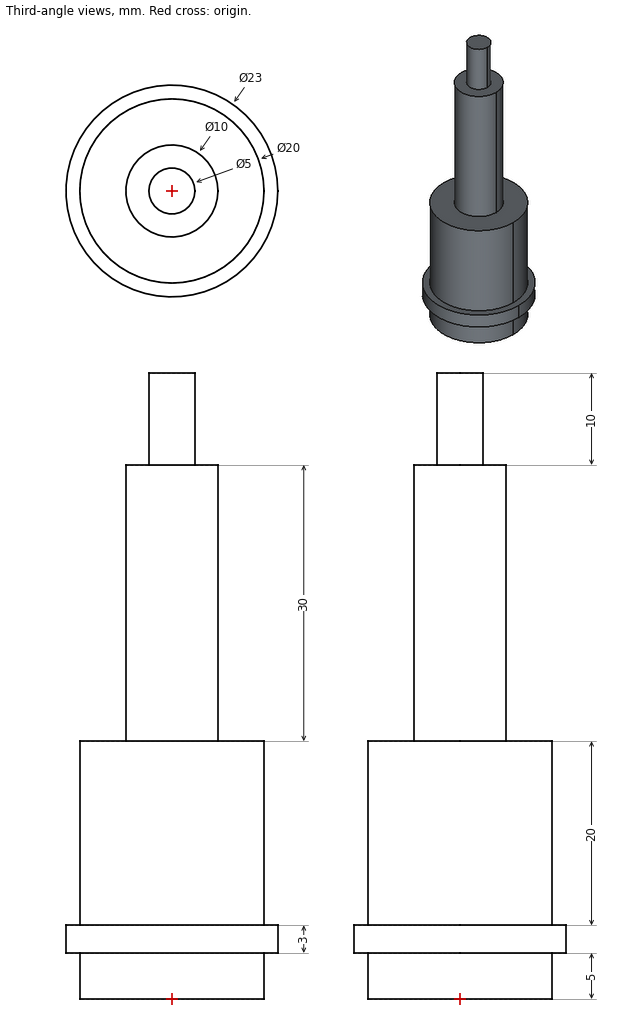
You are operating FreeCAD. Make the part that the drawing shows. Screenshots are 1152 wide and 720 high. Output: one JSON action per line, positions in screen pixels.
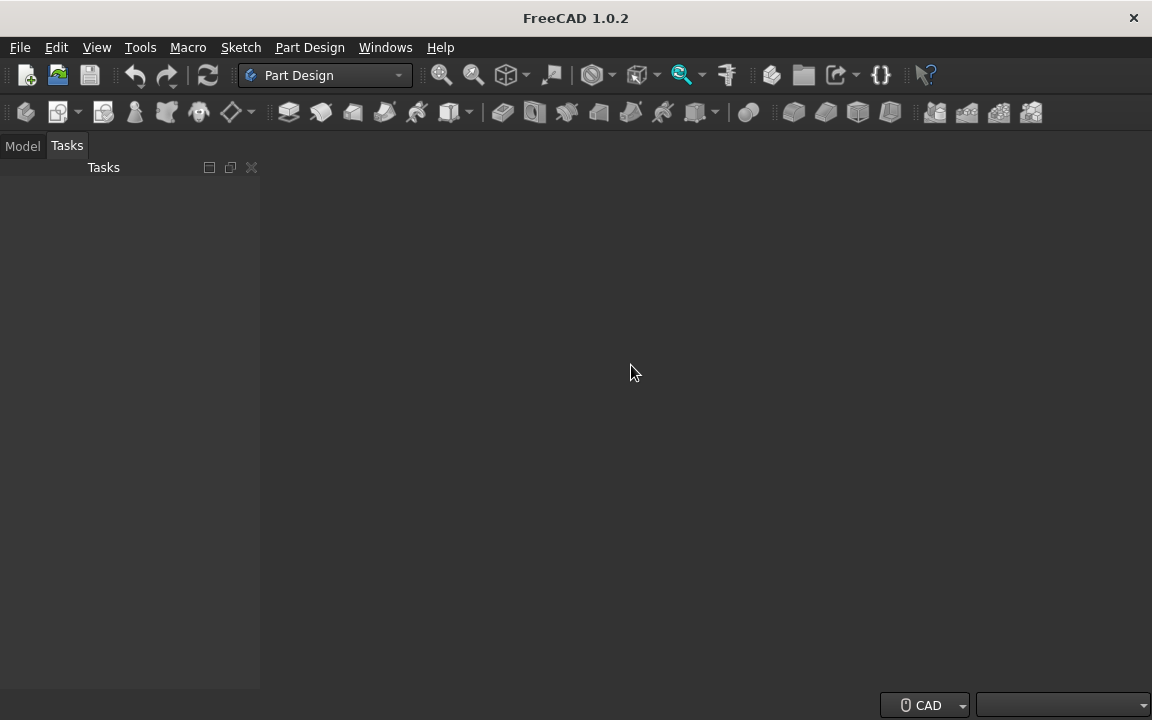
{"action": "left_click", "coordinate": [26, 76]}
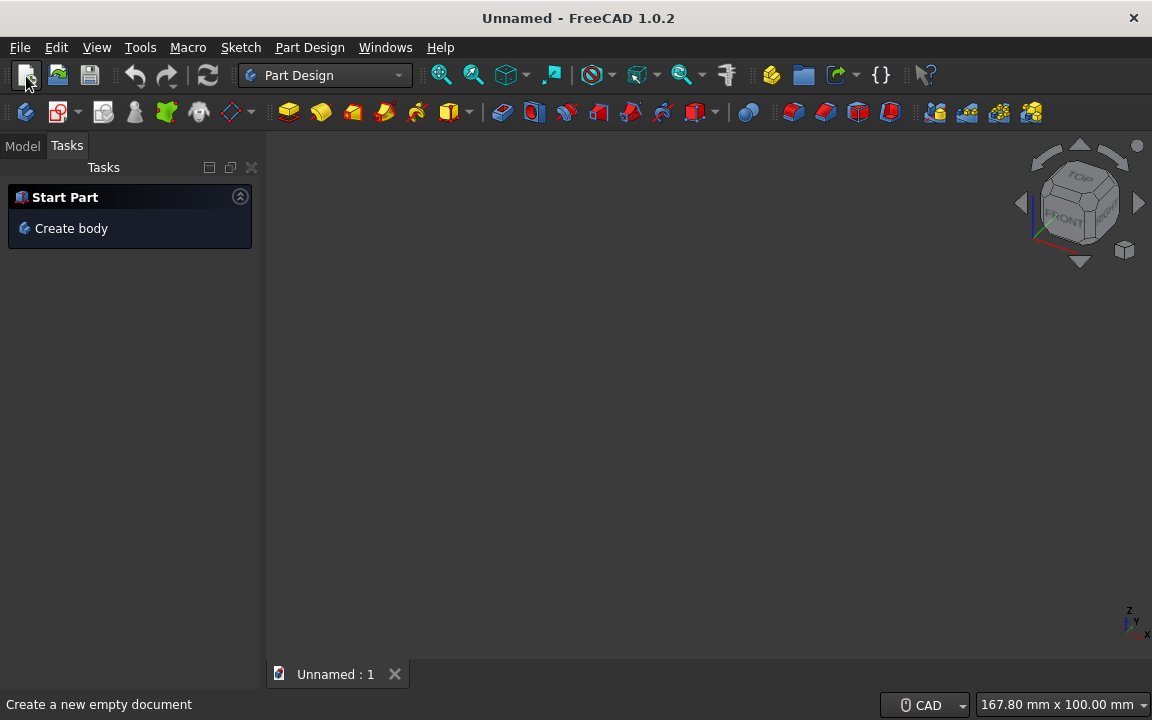
{"action": "left_click", "coordinate": [58, 112]}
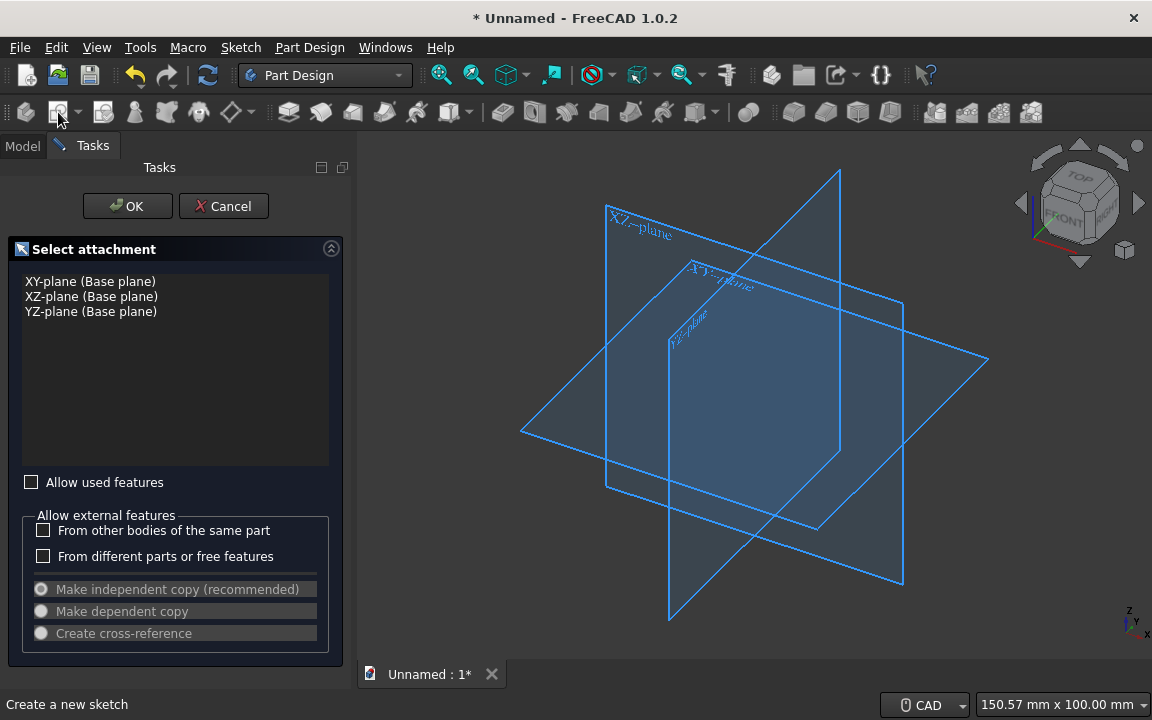
{"action": "left_click", "coordinate": [82, 282]}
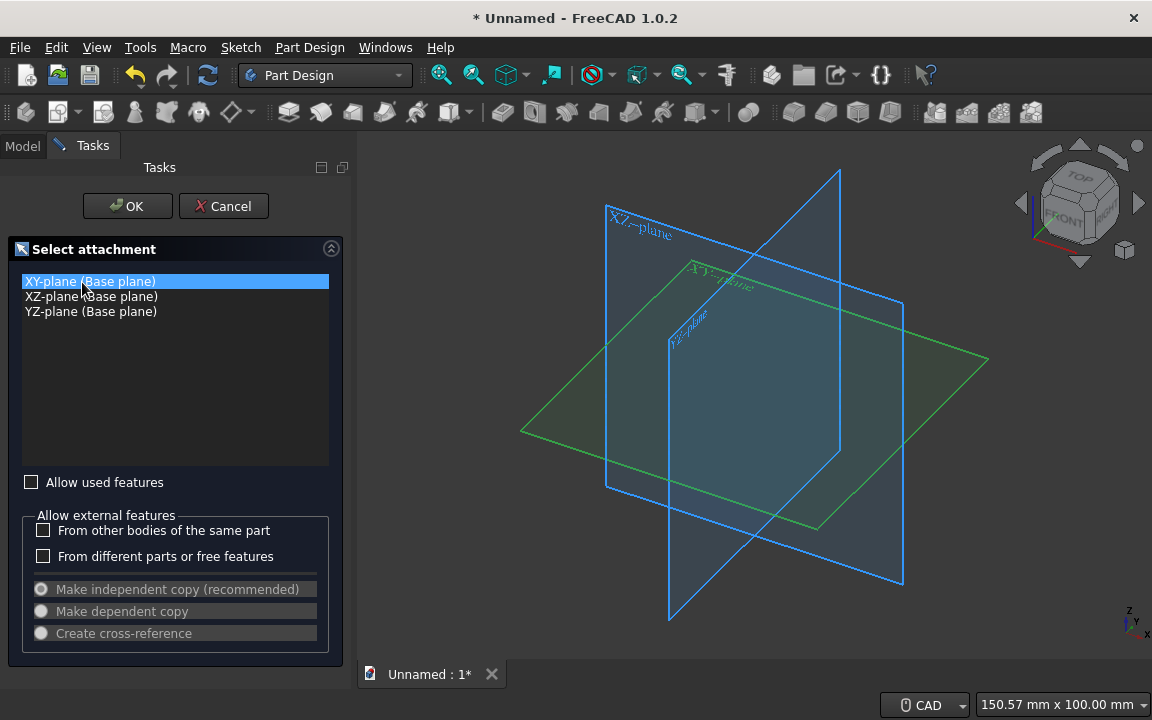
{"action": "left_click", "coordinate": [128, 206]}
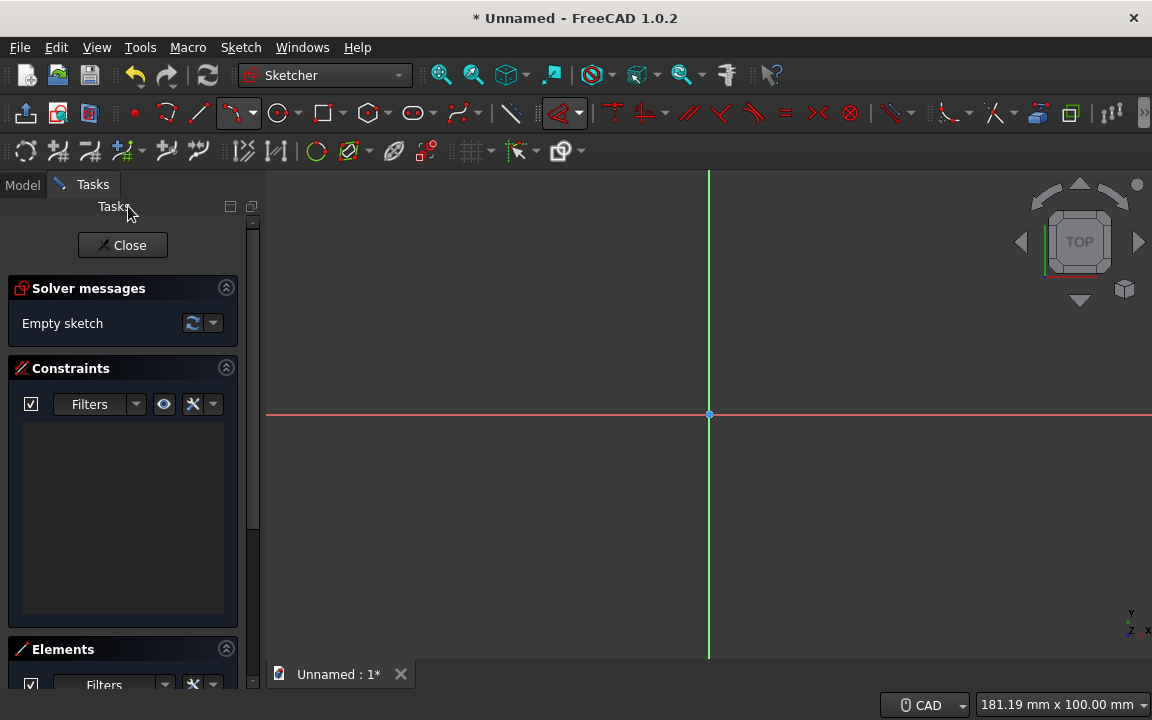
{"action": "scroll", "coordinate": [739, 415], "scroll_direction": "up", "scroll_amount": 6}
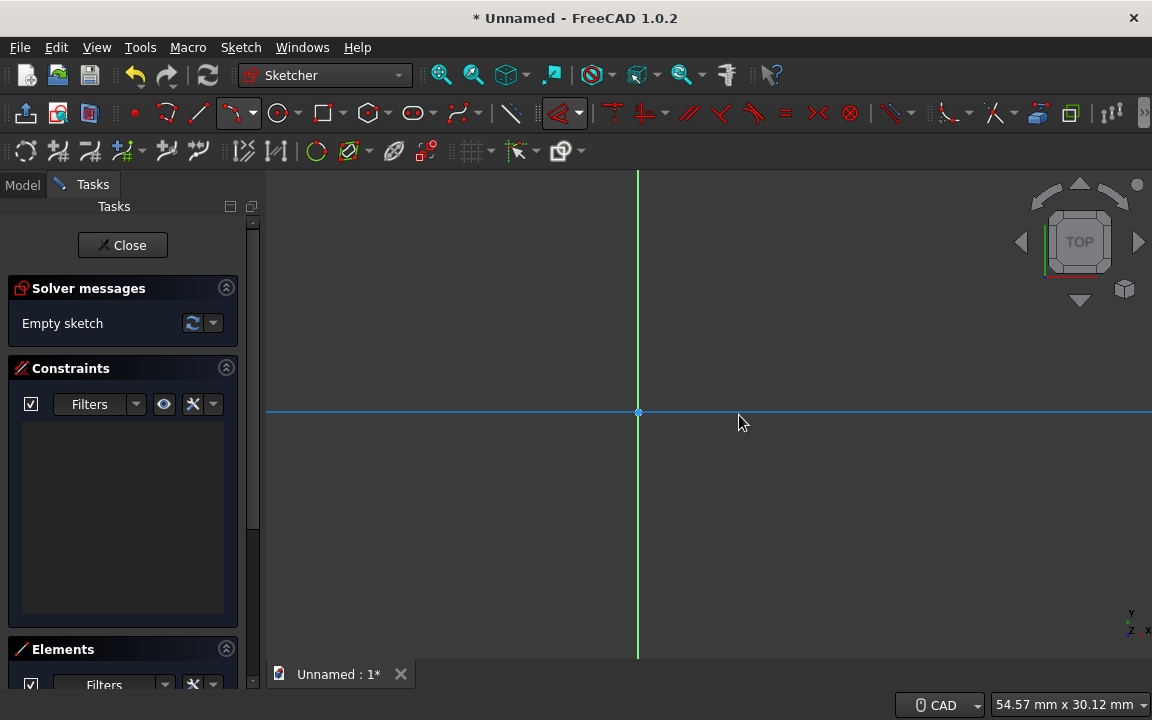
{"action": "left_click", "coordinate": [278, 114]}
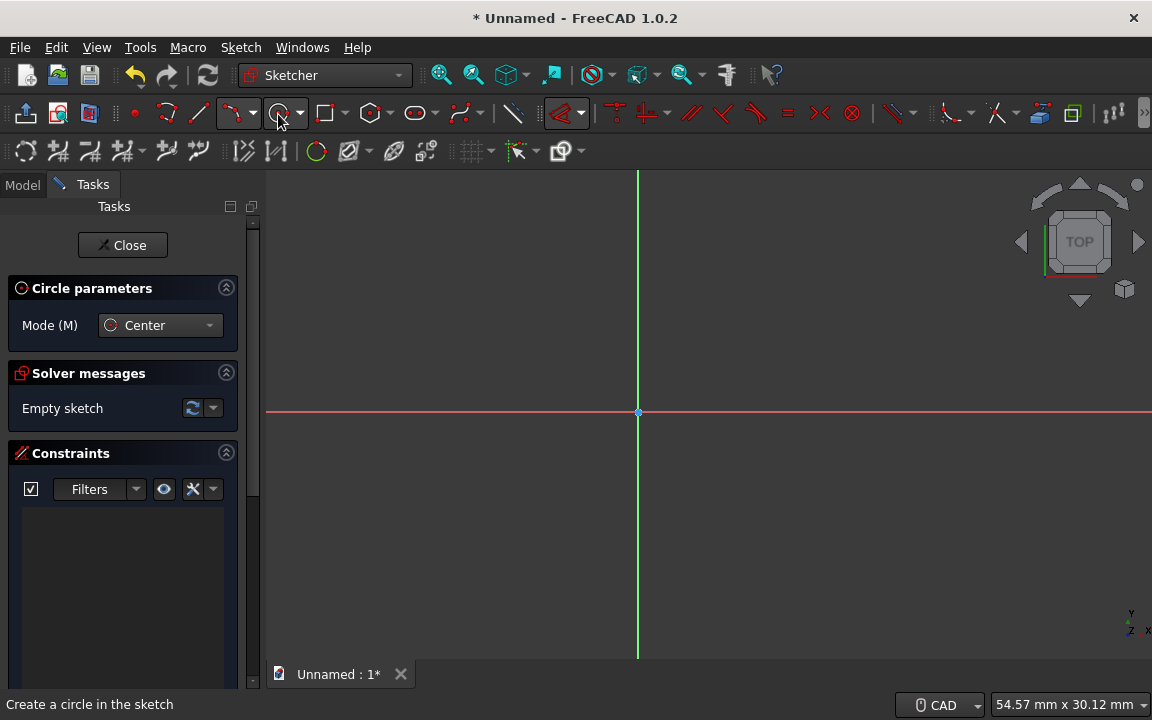
{"action": "left_click", "coordinate": [638, 412]}
{"action": "mouse_move", "coordinate": [753, 297]}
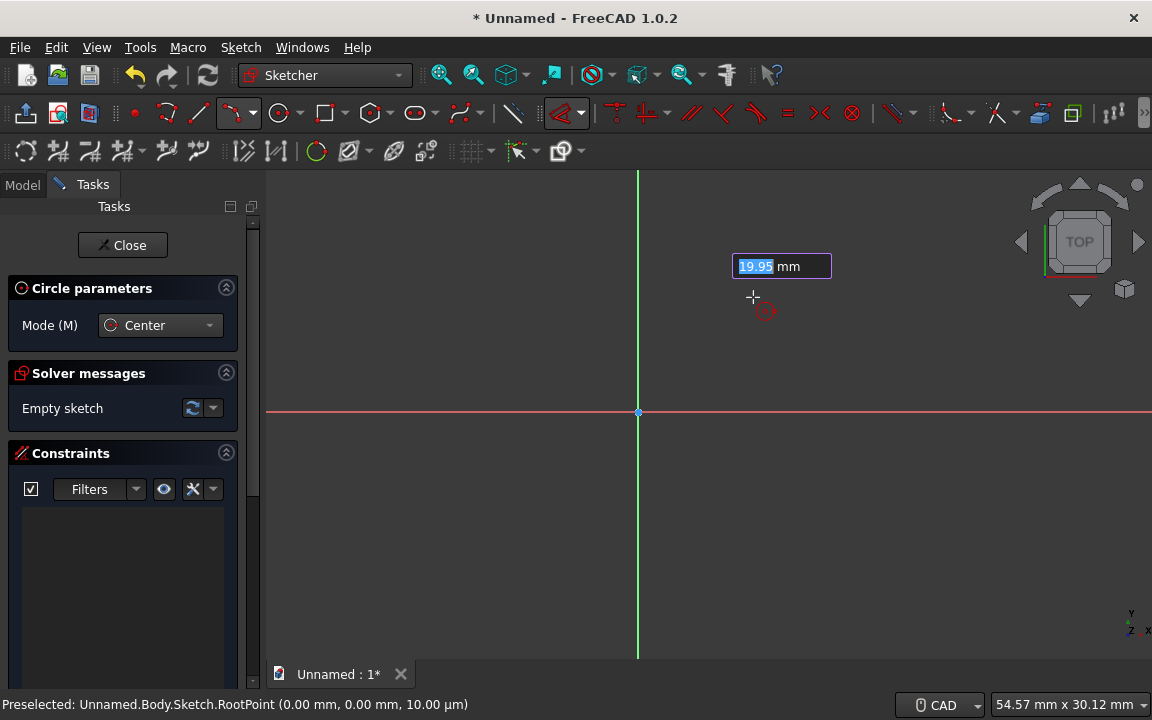
{"action": "type", "text": "20"}
{"action": "key", "text": "Return"}
{"action": "key", "text": "Escape"}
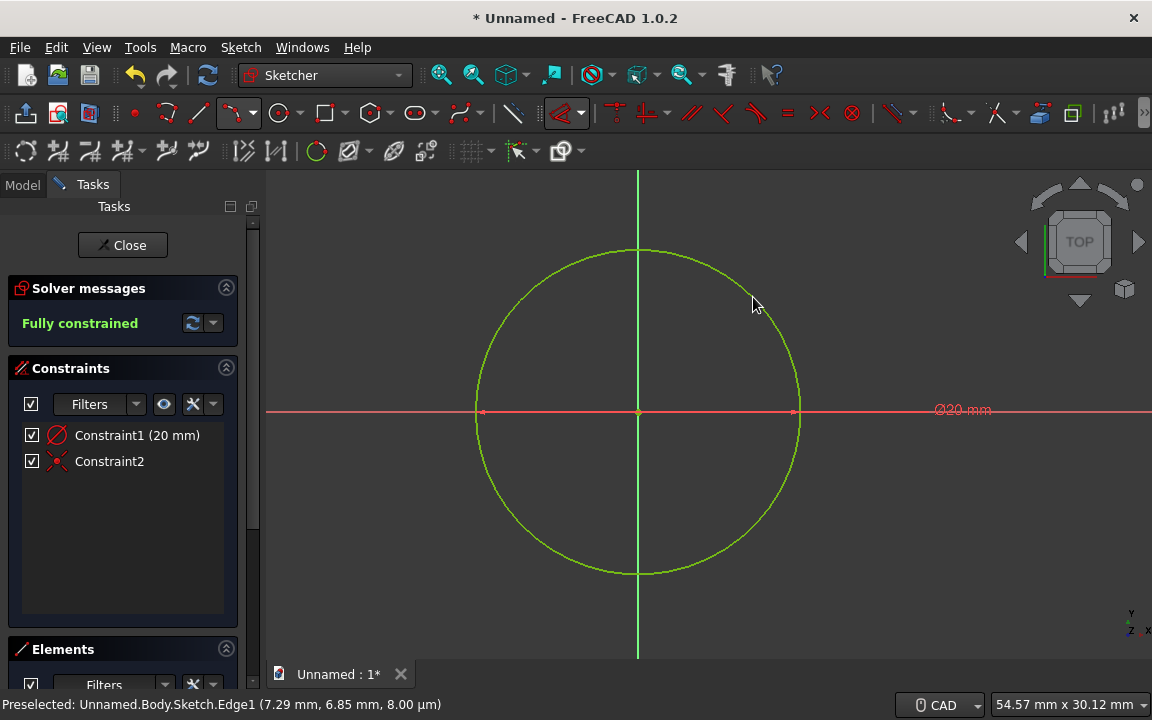
{"action": "left_click", "coordinate": [123, 245]}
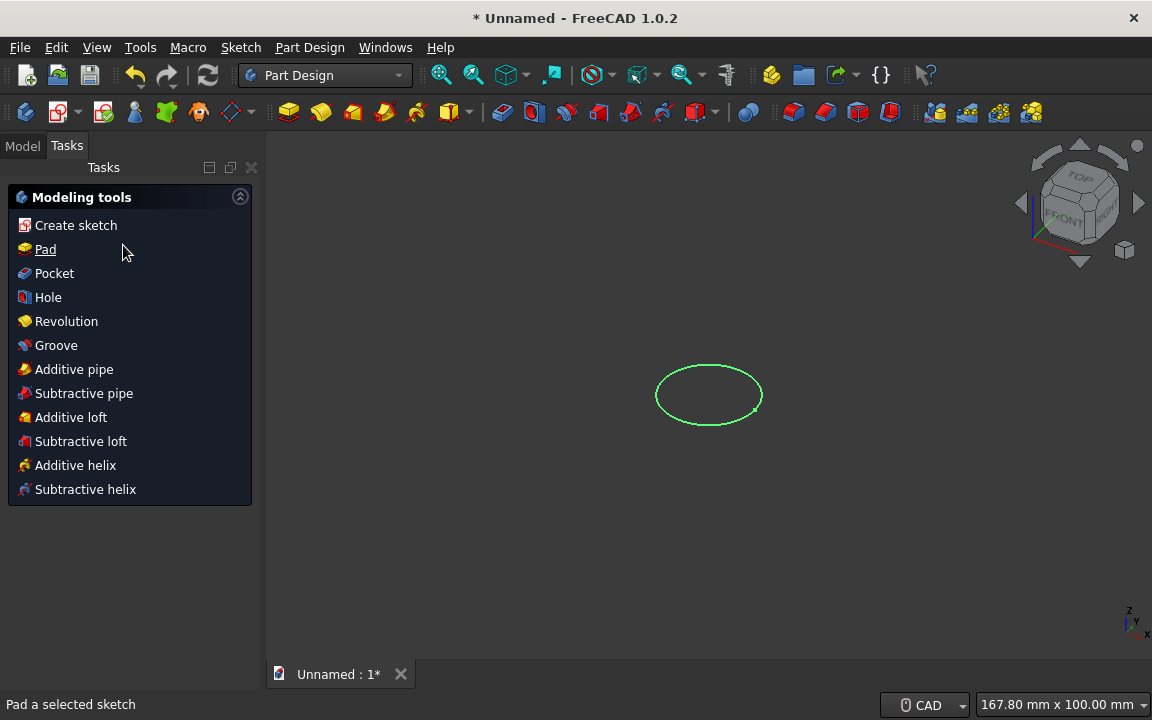
{"action": "left_click", "coordinate": [290, 112]}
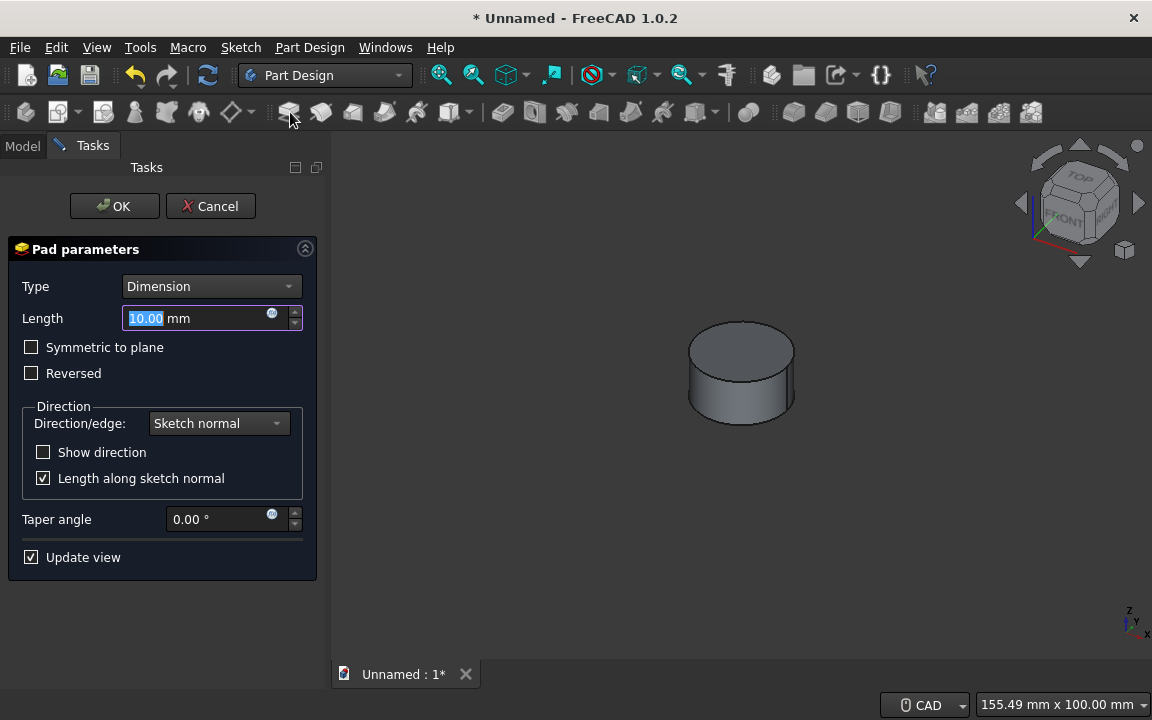
{"action": "type", "text": "5"}
{"action": "key", "text": "Tab"}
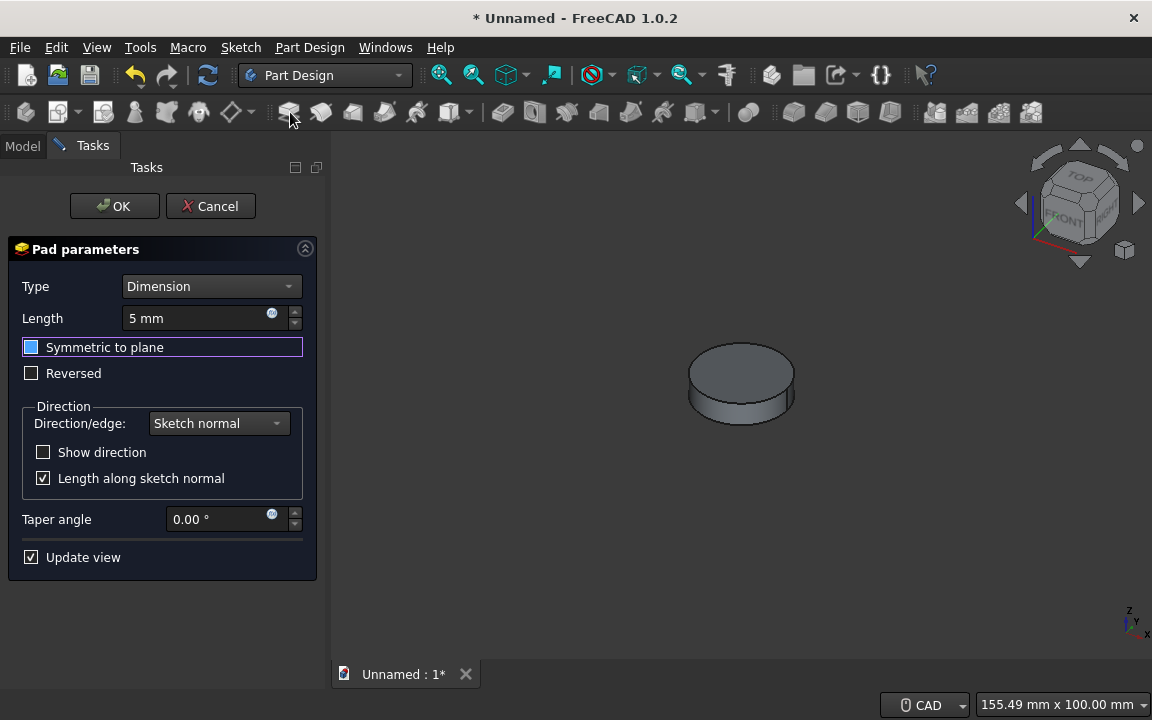
{"action": "left_click", "coordinate": [115, 206]}